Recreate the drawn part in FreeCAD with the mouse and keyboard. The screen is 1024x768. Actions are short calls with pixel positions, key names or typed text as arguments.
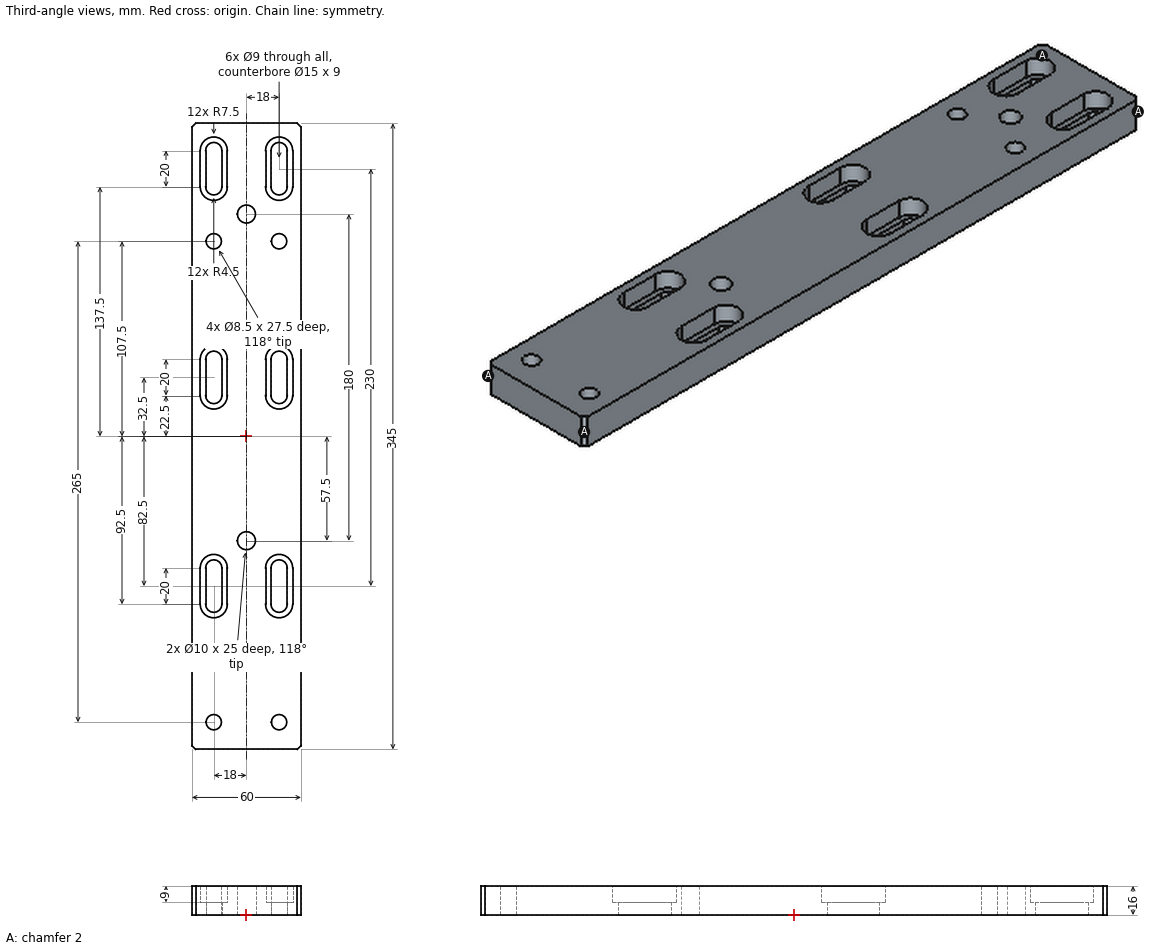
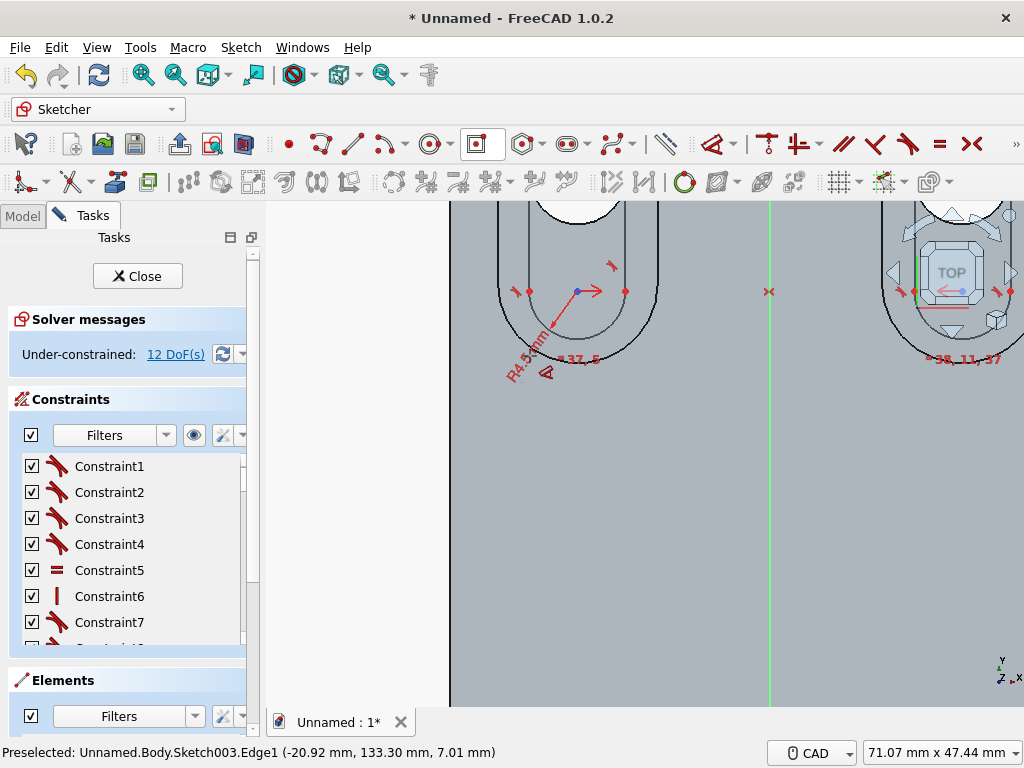
scroll(552, 336, down, 11)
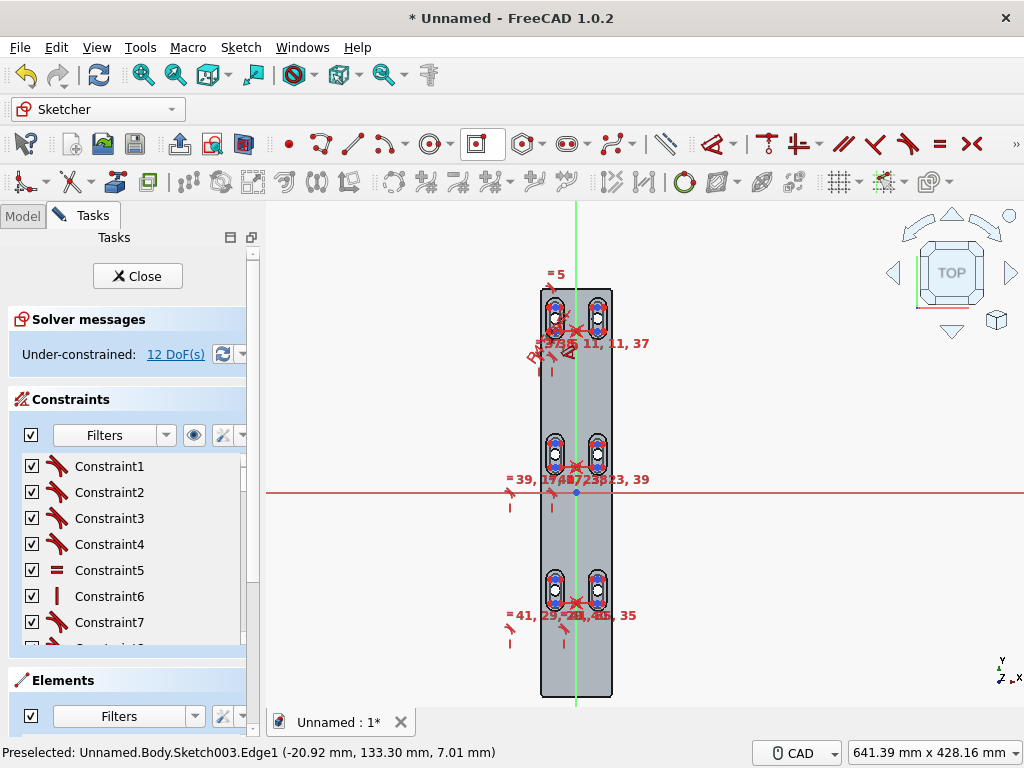
scroll(550, 326, up, 6)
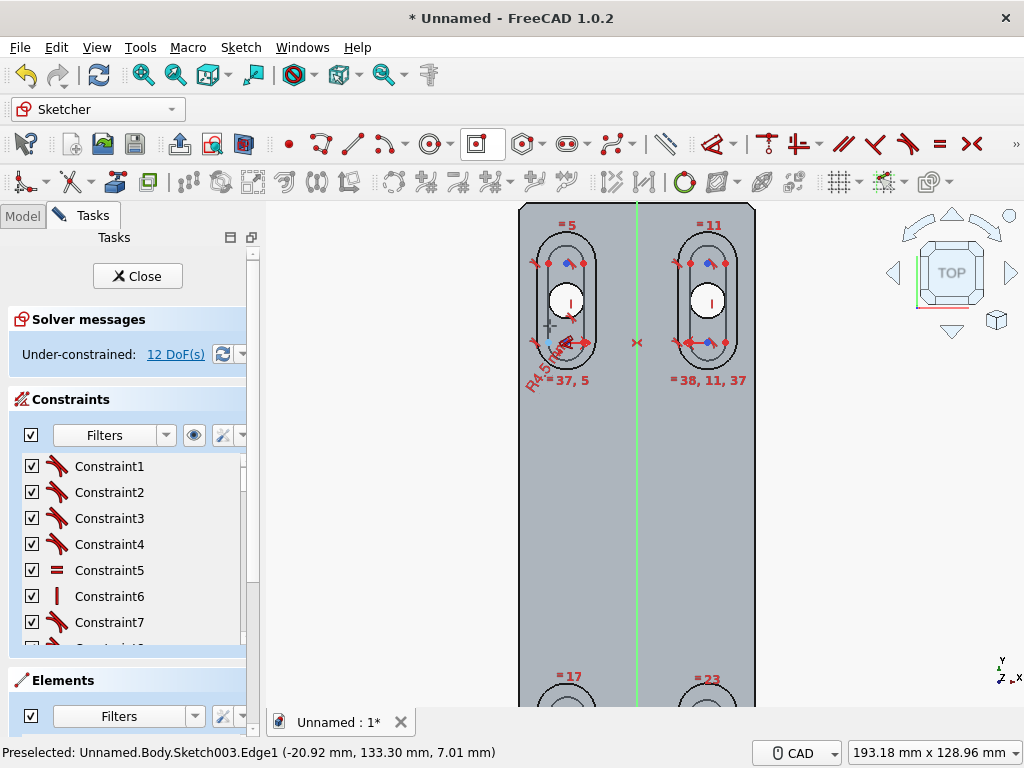
click(548, 327)
click(514, 303)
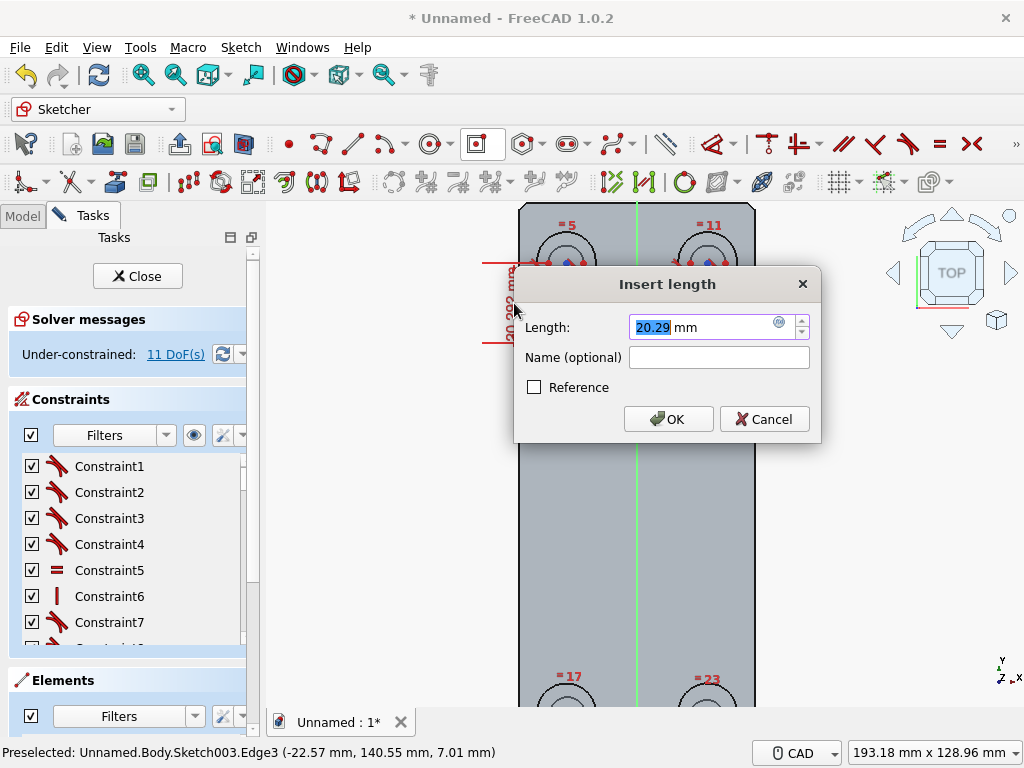
text(20)
key(Return)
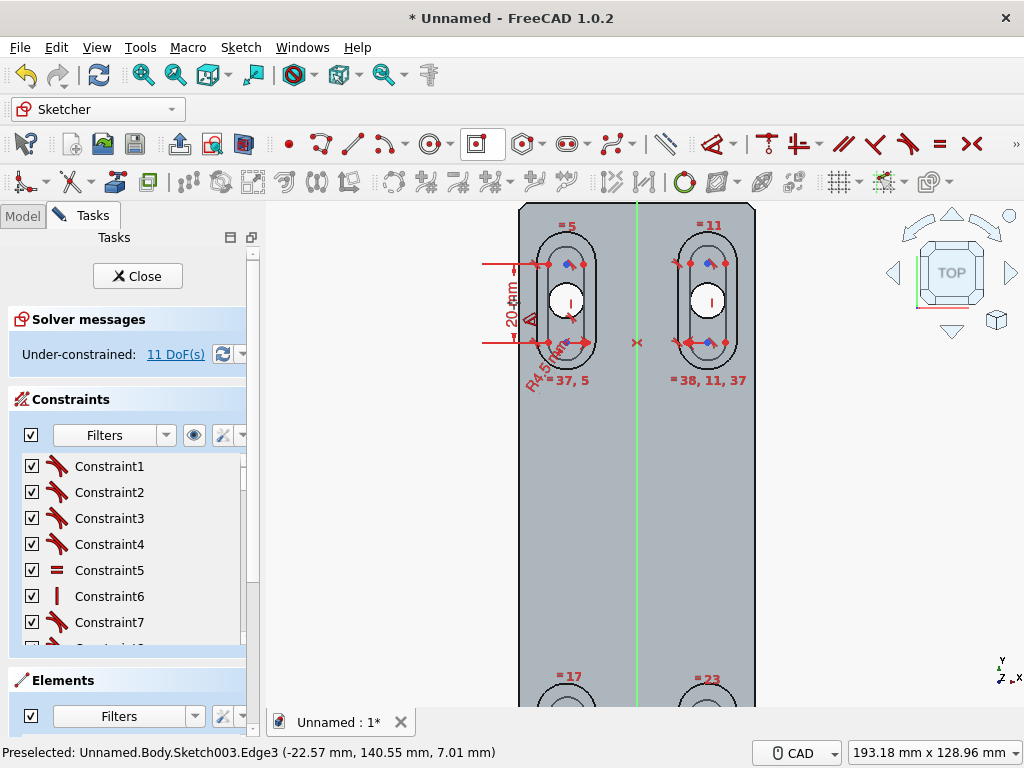
click(690, 319)
click(656, 303)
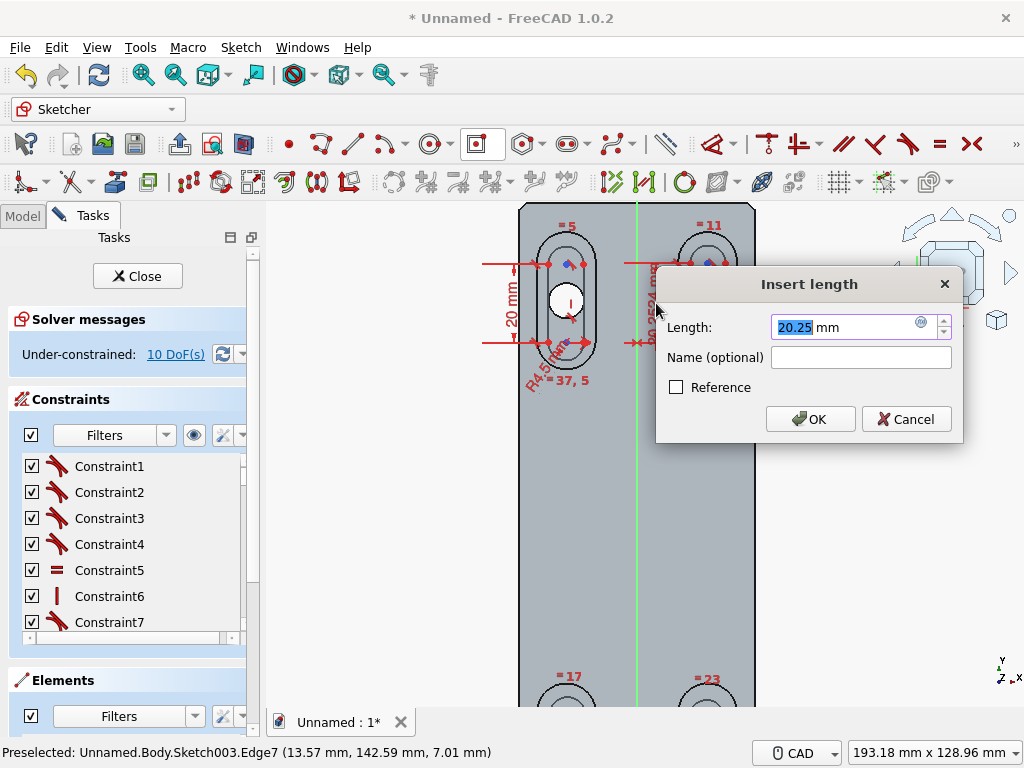
text(20)
key(Return)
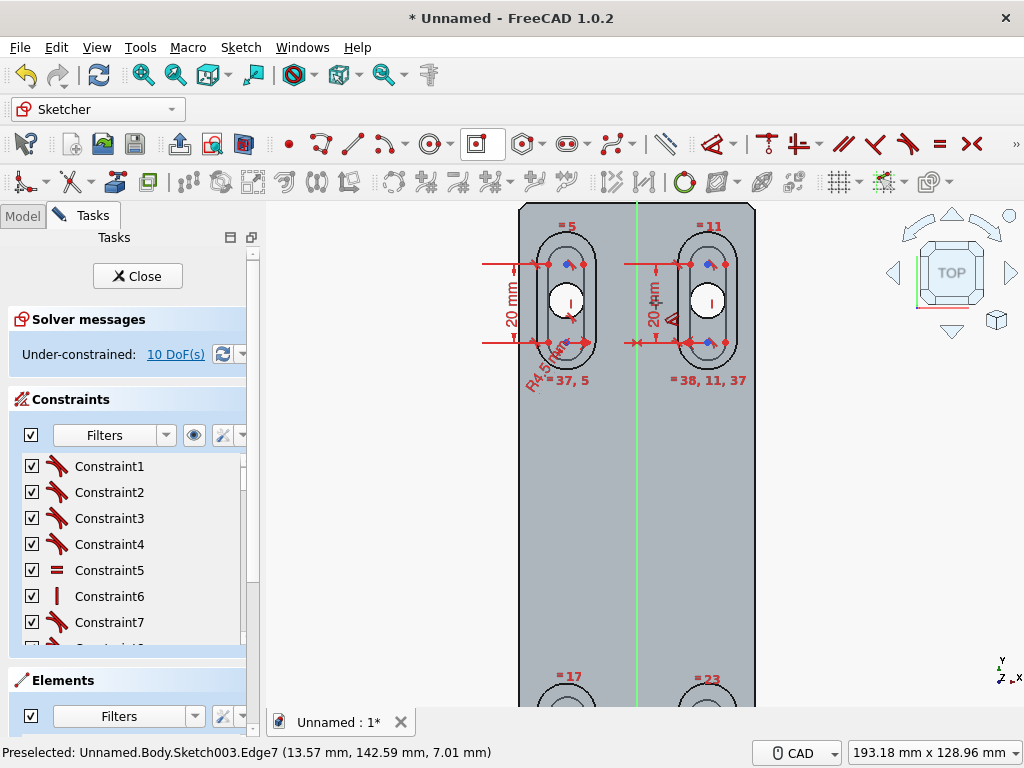
scroll(550, 326, down, 6)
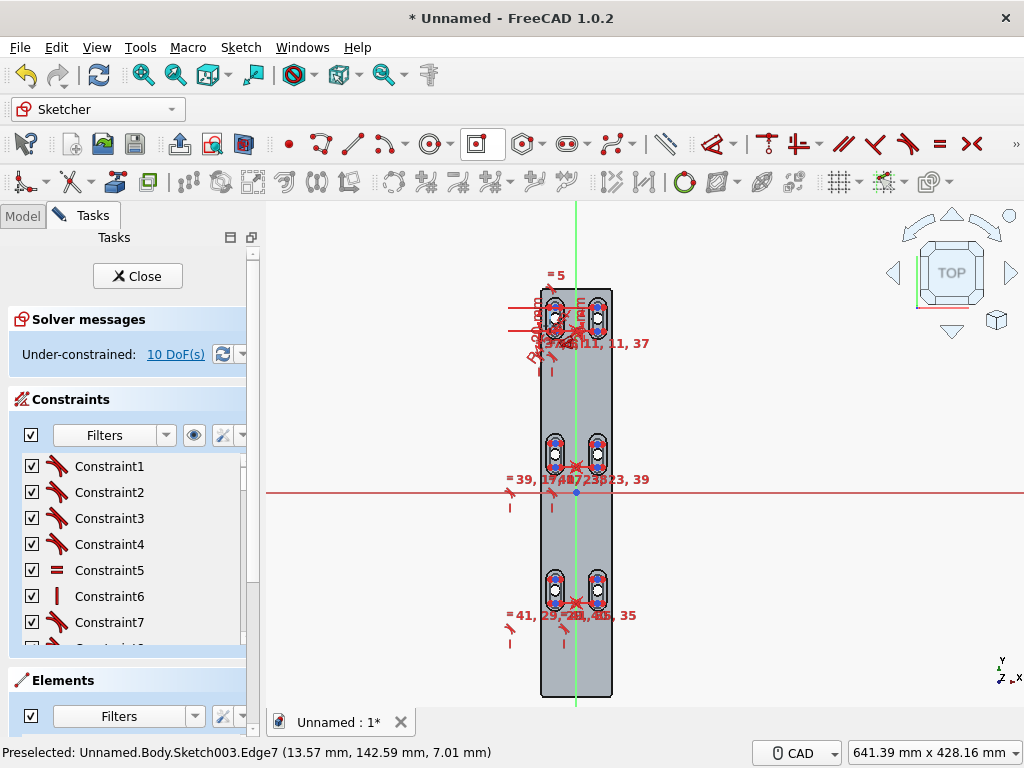
scroll(550, 460, up, 4)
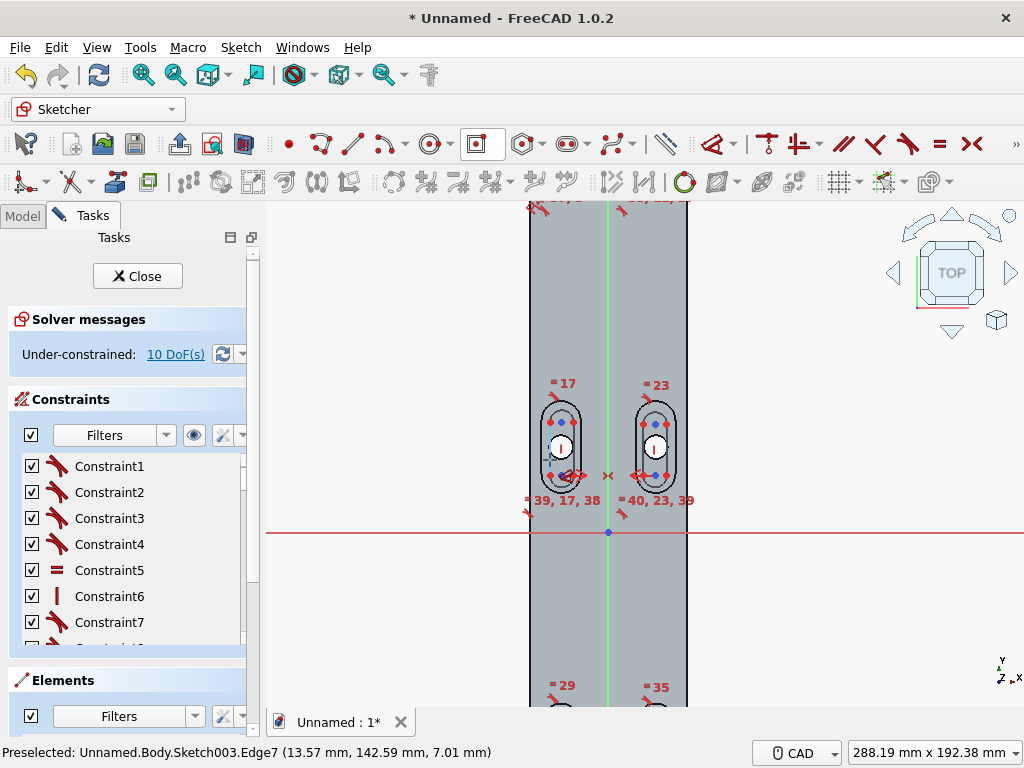
click(550, 460)
click(516, 449)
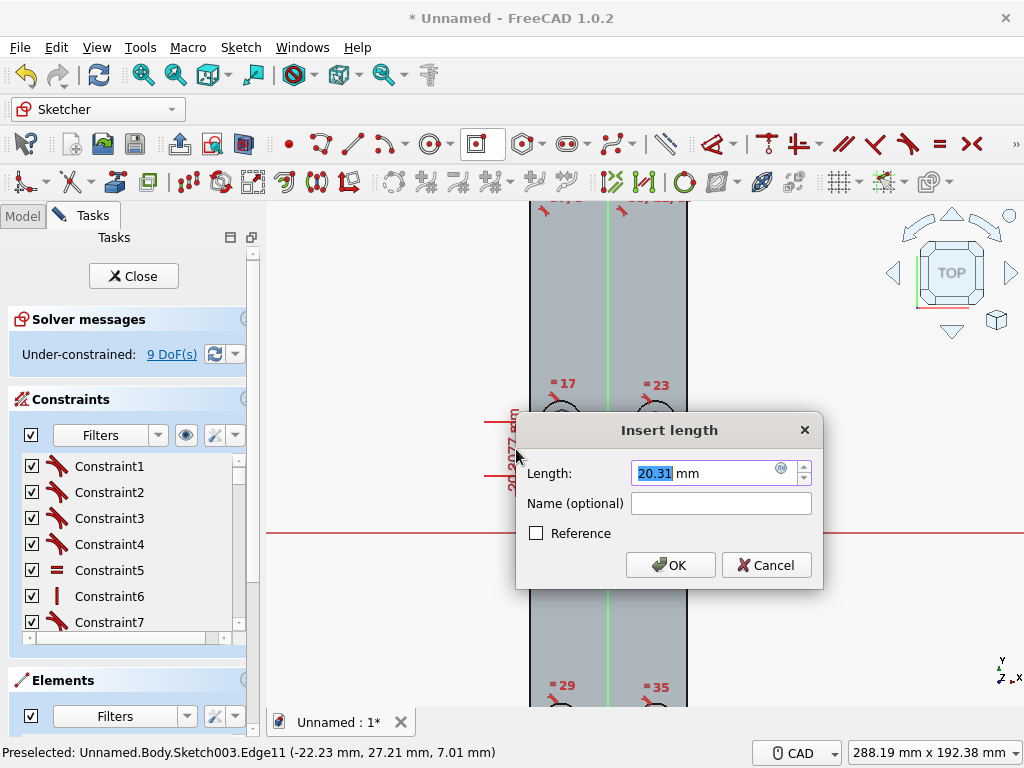
text(20)
key(Return)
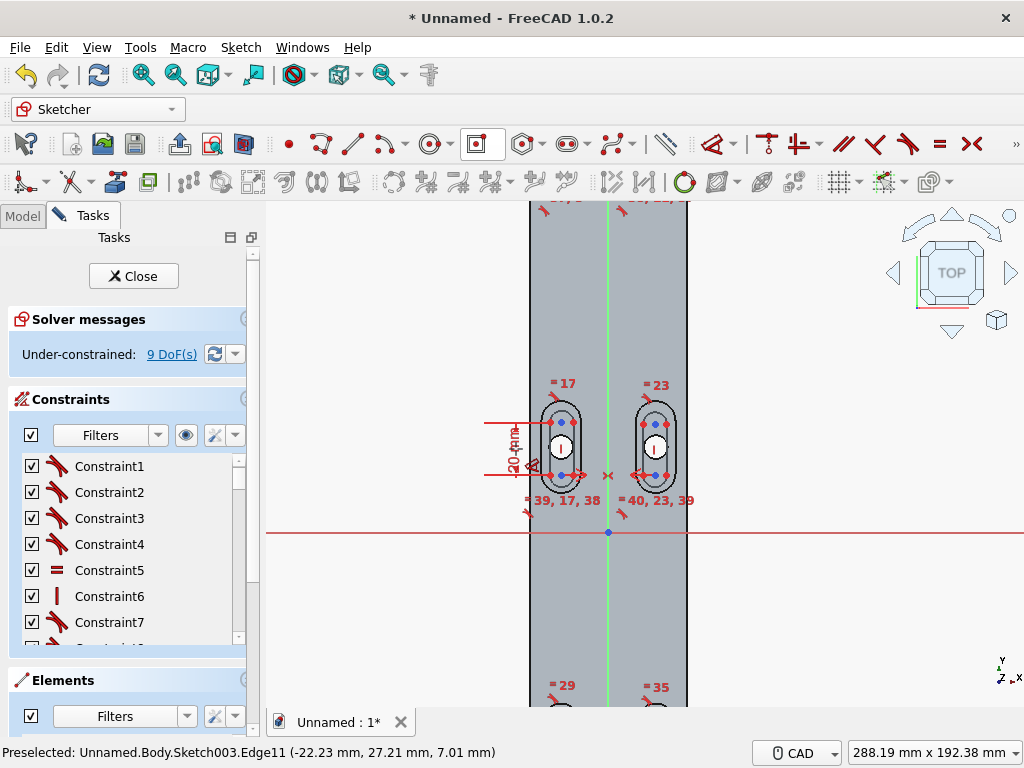
click(643, 460)
click(701, 450)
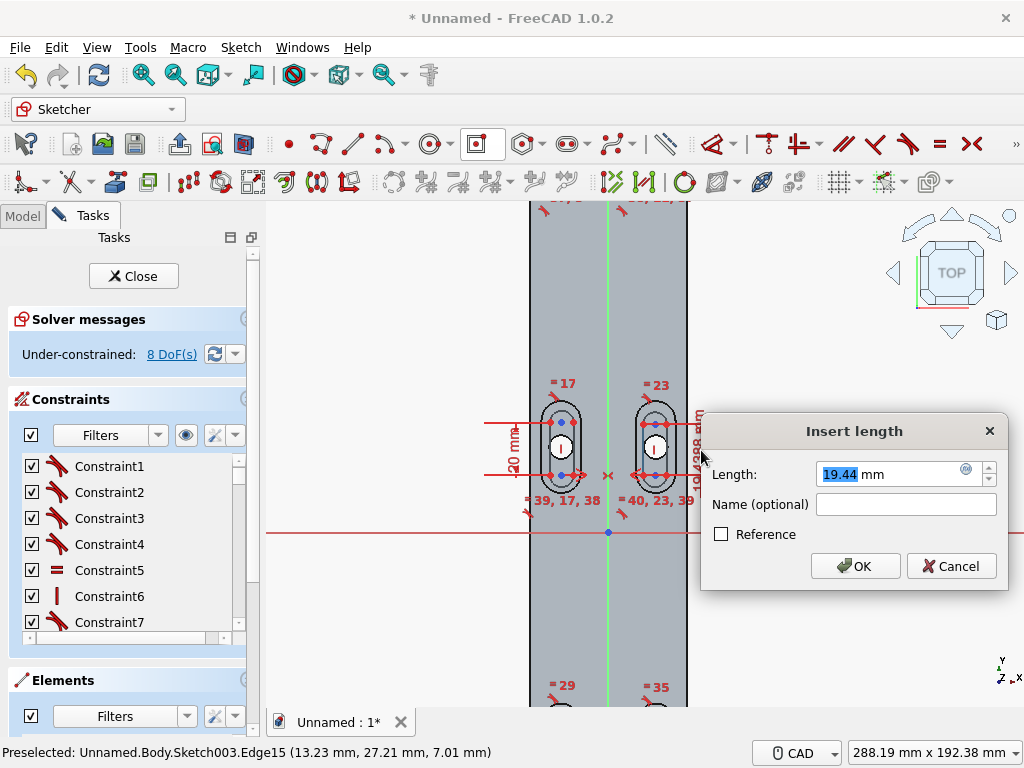
text(20)
key(Return)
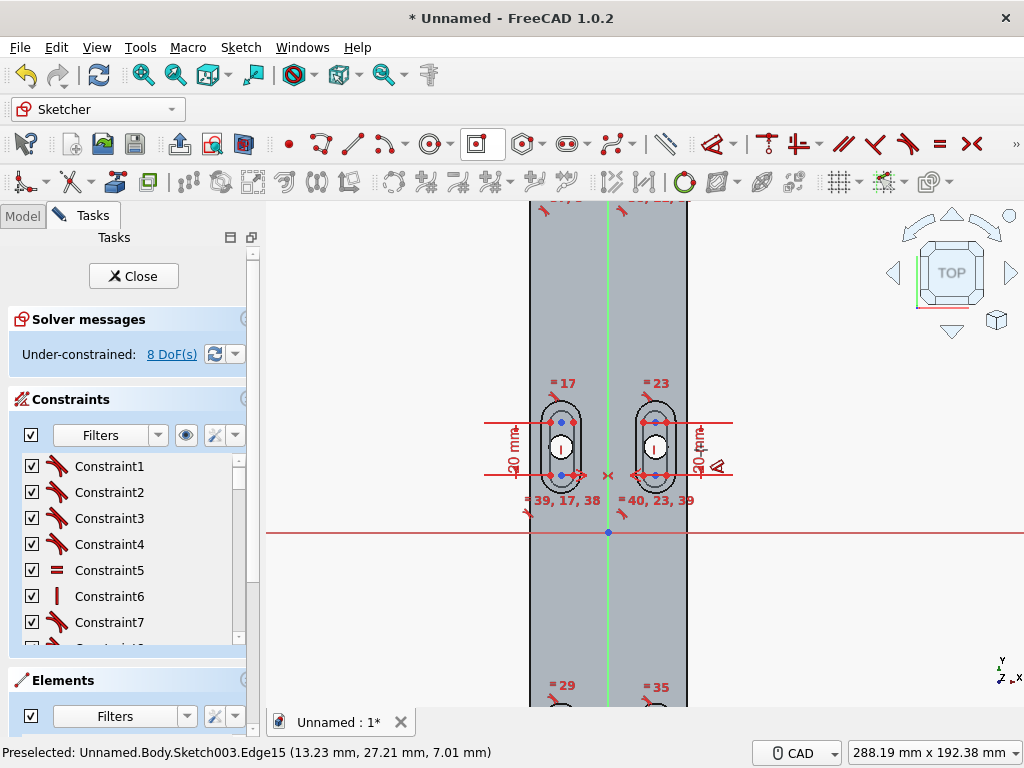
scroll(550, 460, down, 4)